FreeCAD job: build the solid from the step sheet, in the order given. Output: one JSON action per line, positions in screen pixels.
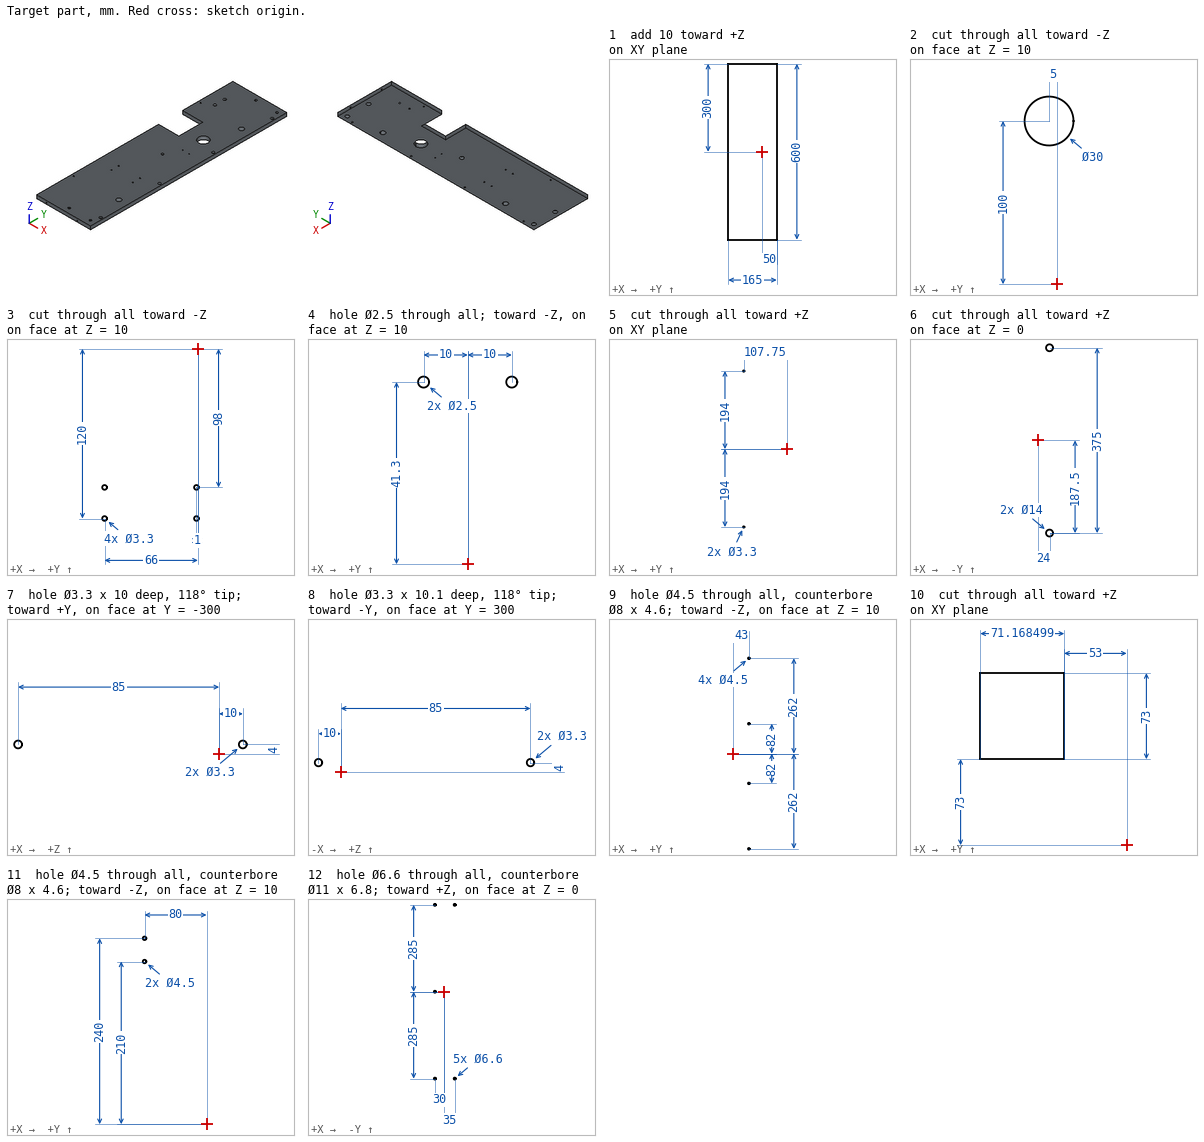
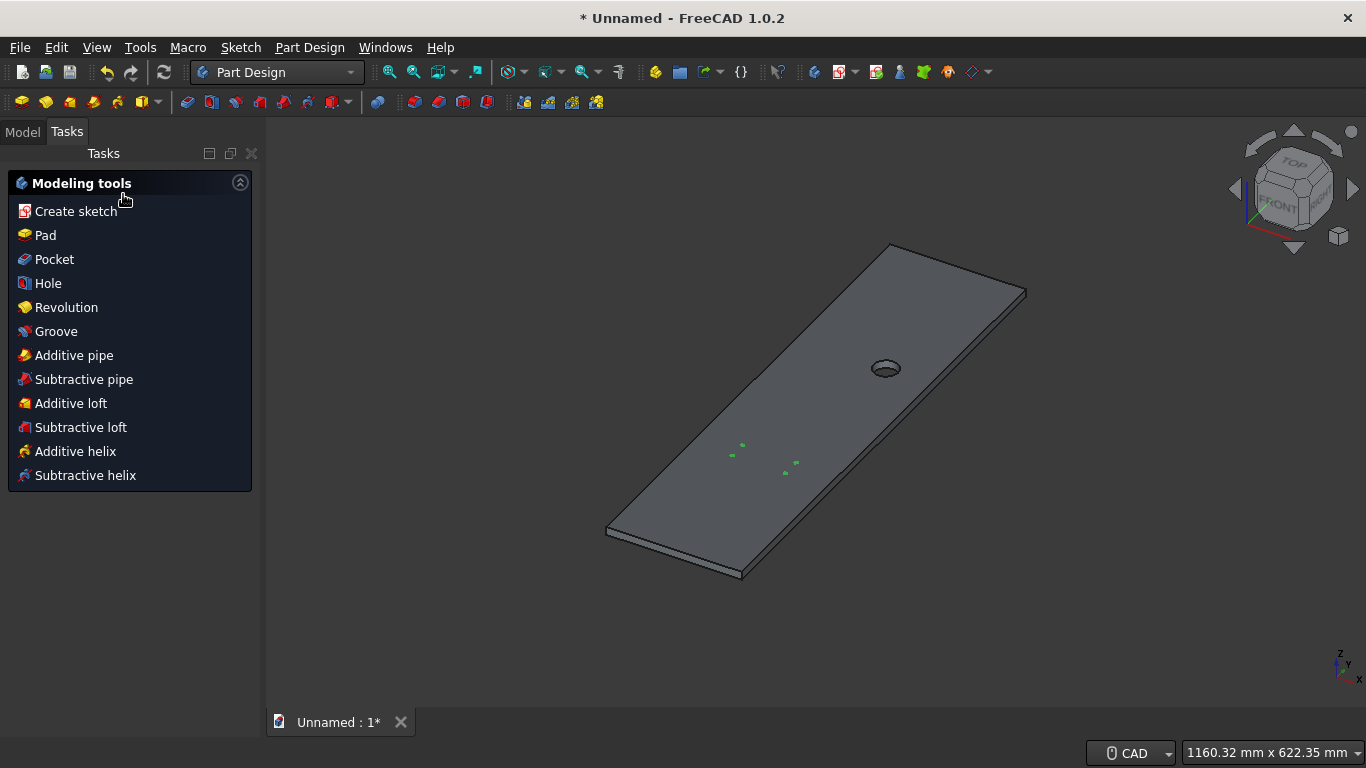
{"action": "left_click", "coordinate": [188, 102]}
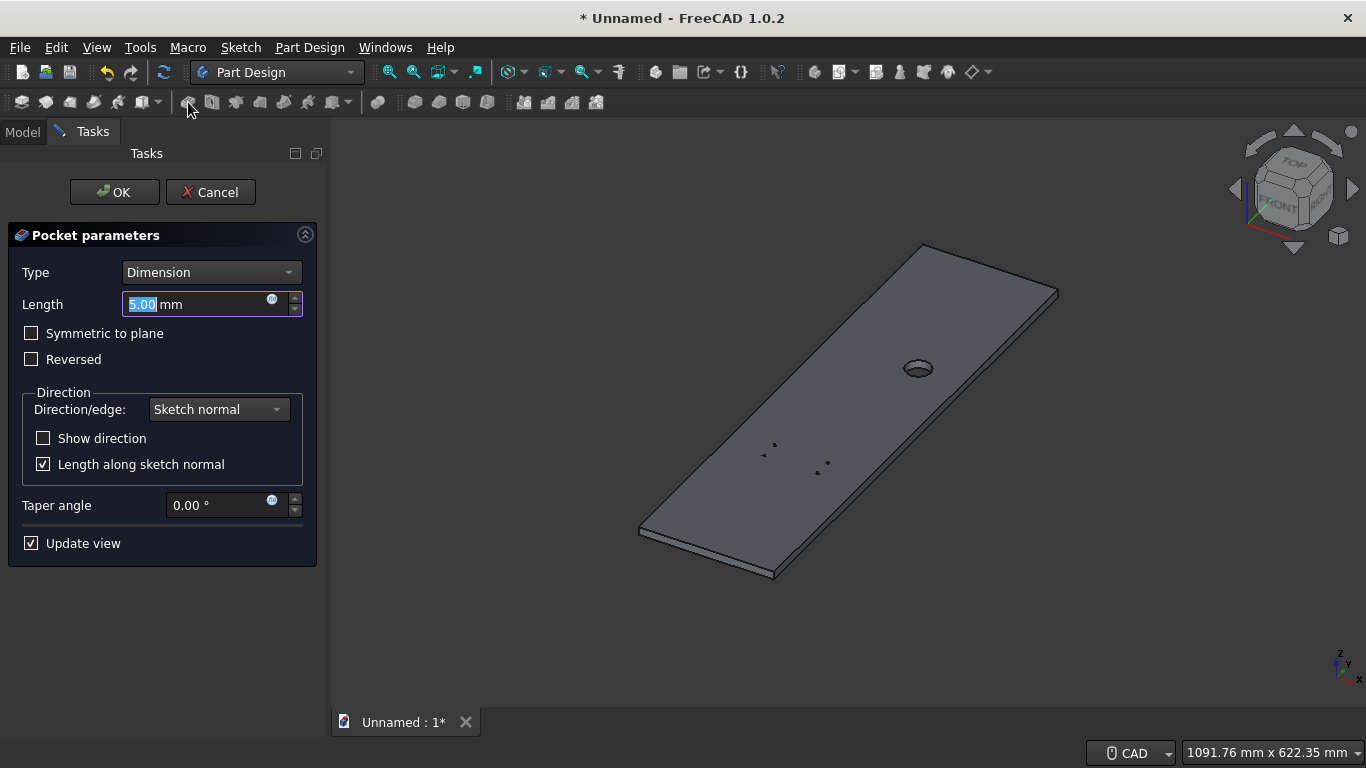
{"action": "left_click", "coordinate": [212, 272]}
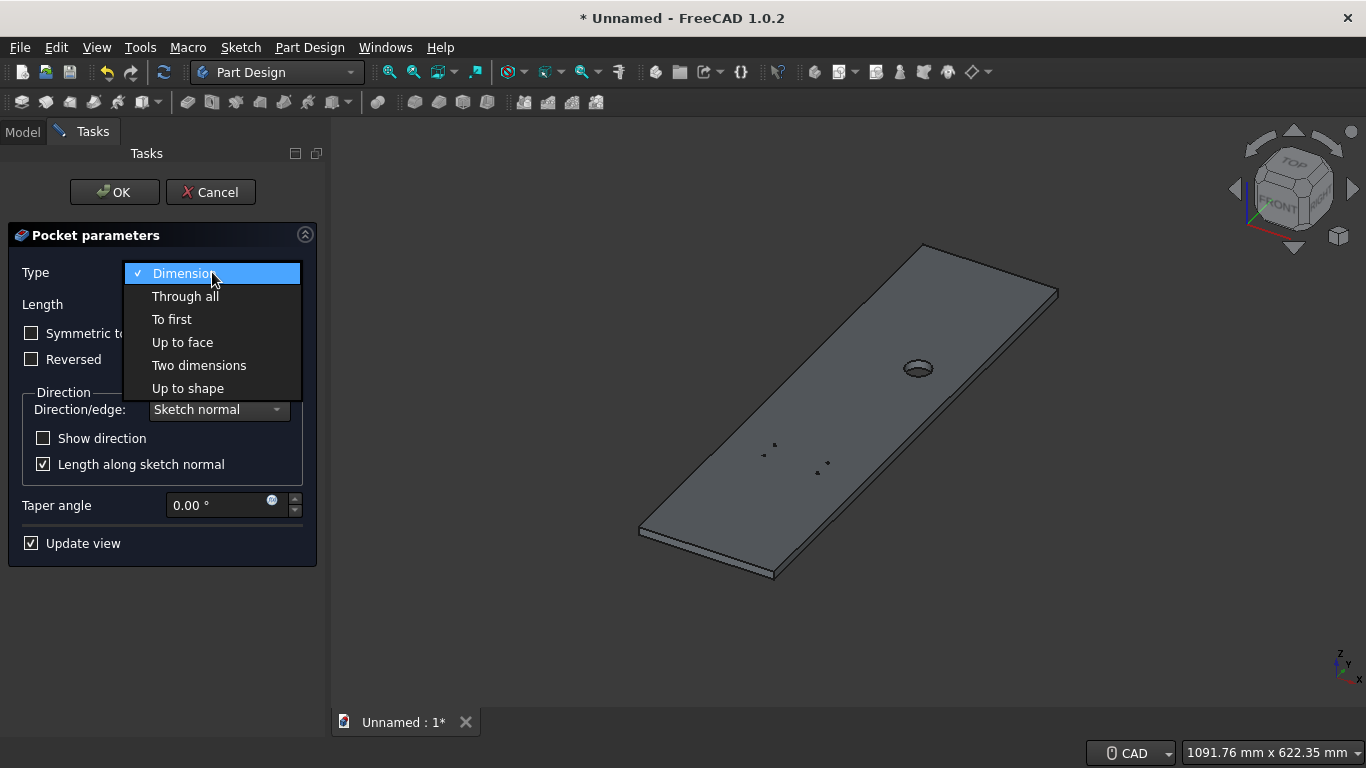
{"action": "left_click", "coordinate": [212, 296]}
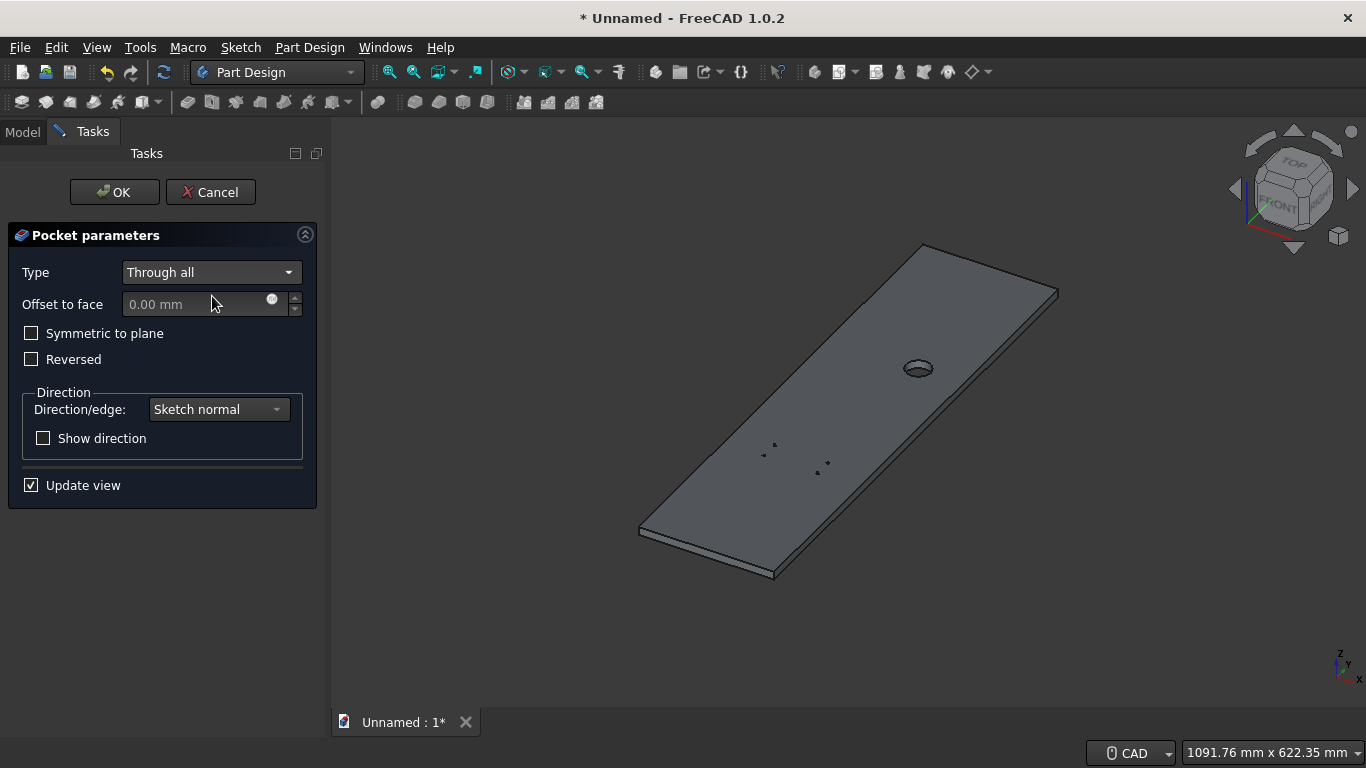
{"action": "left_click", "coordinate": [115, 192]}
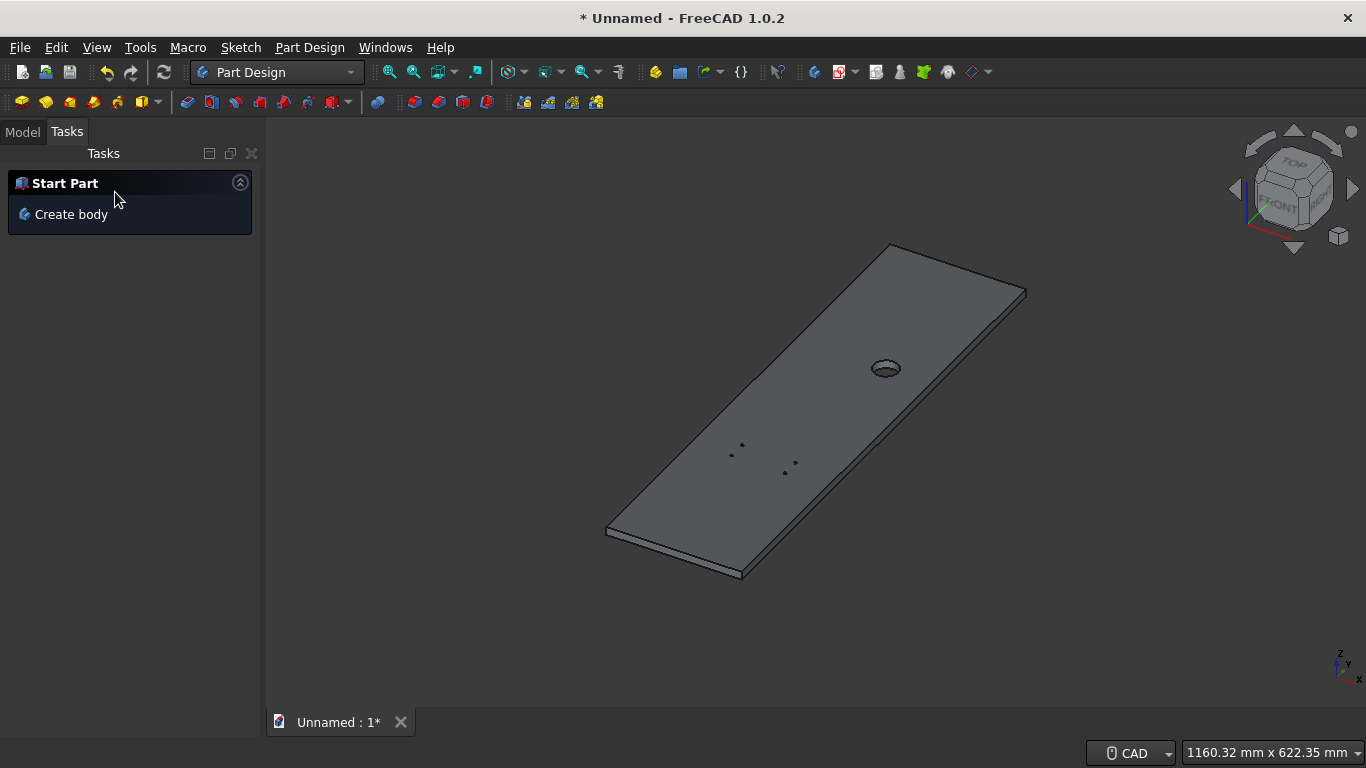
{"action": "left_click", "coordinate": [816, 407]}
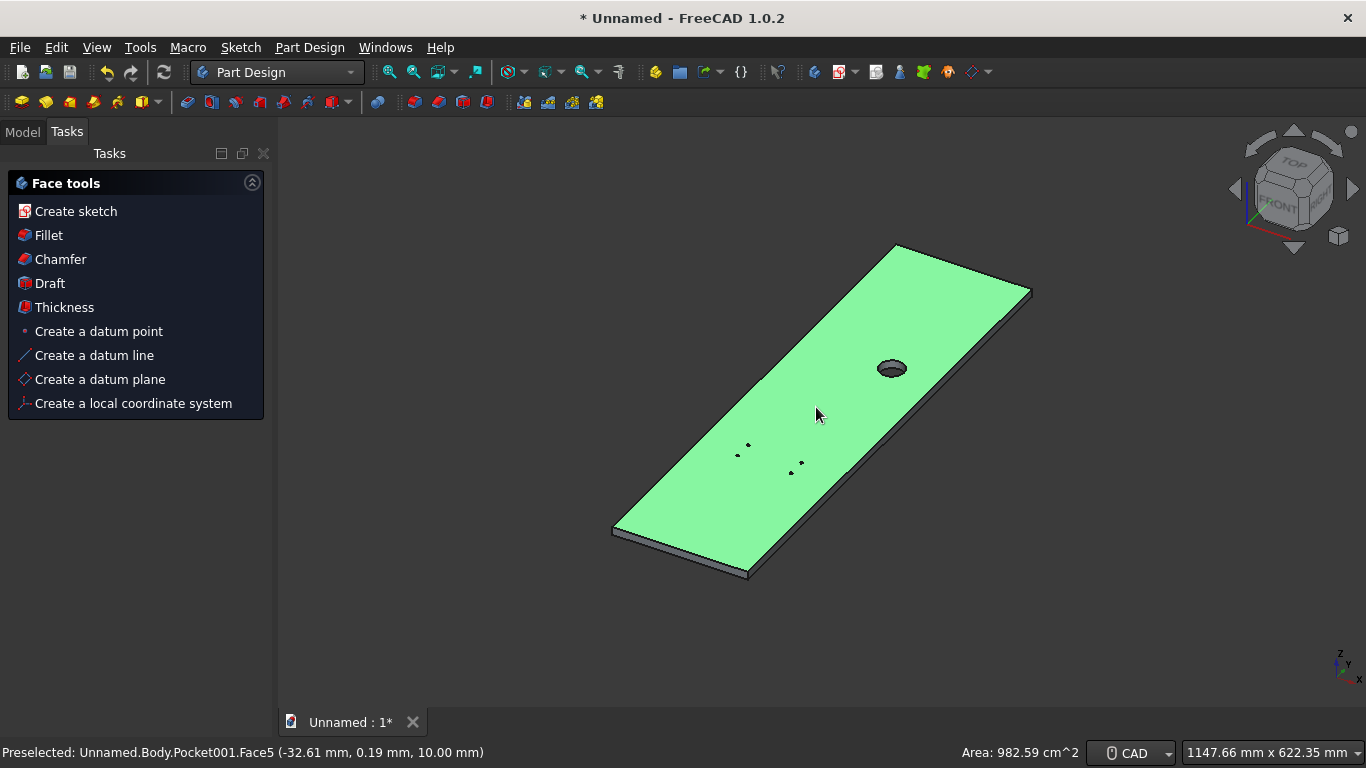
{"action": "left_click", "coordinate": [840, 72]}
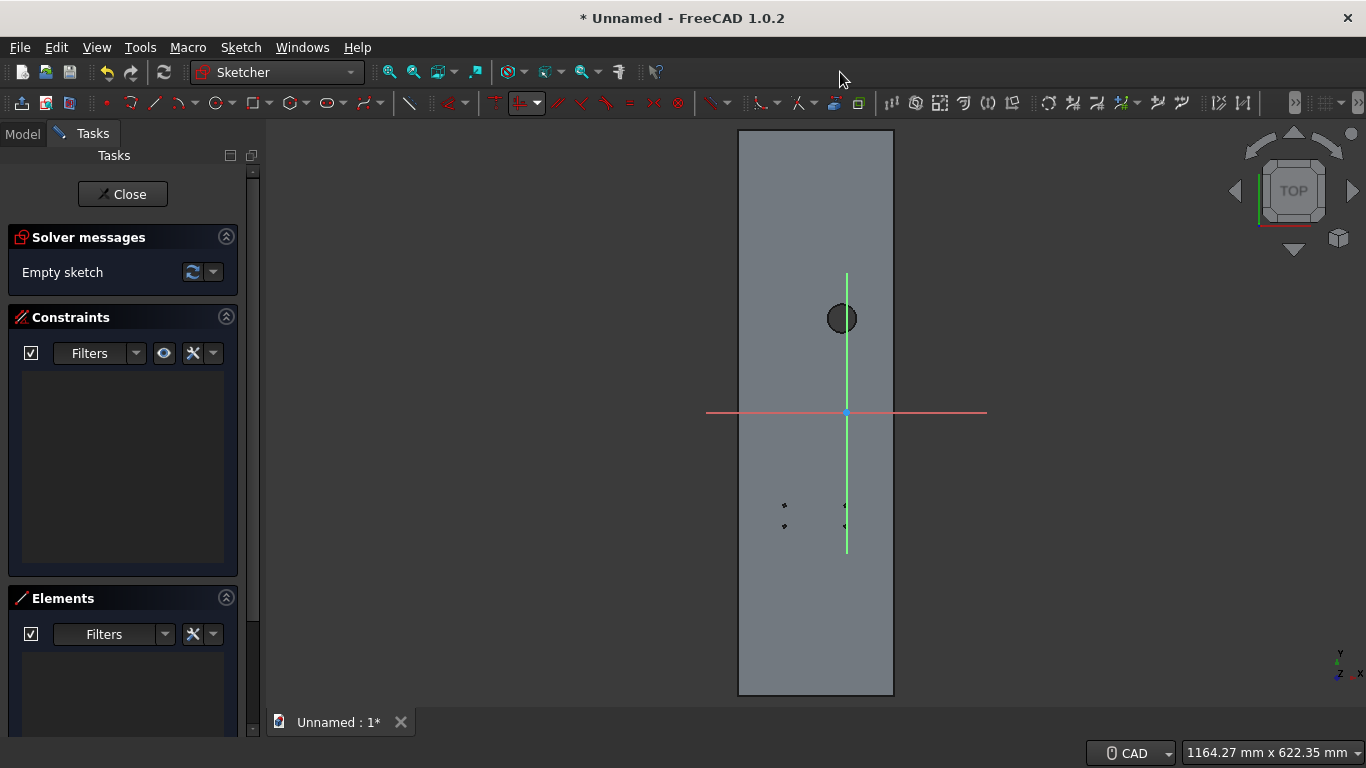
{"action": "scroll", "coordinate": [859, 390], "scroll_direction": "up", "scroll_amount": 11}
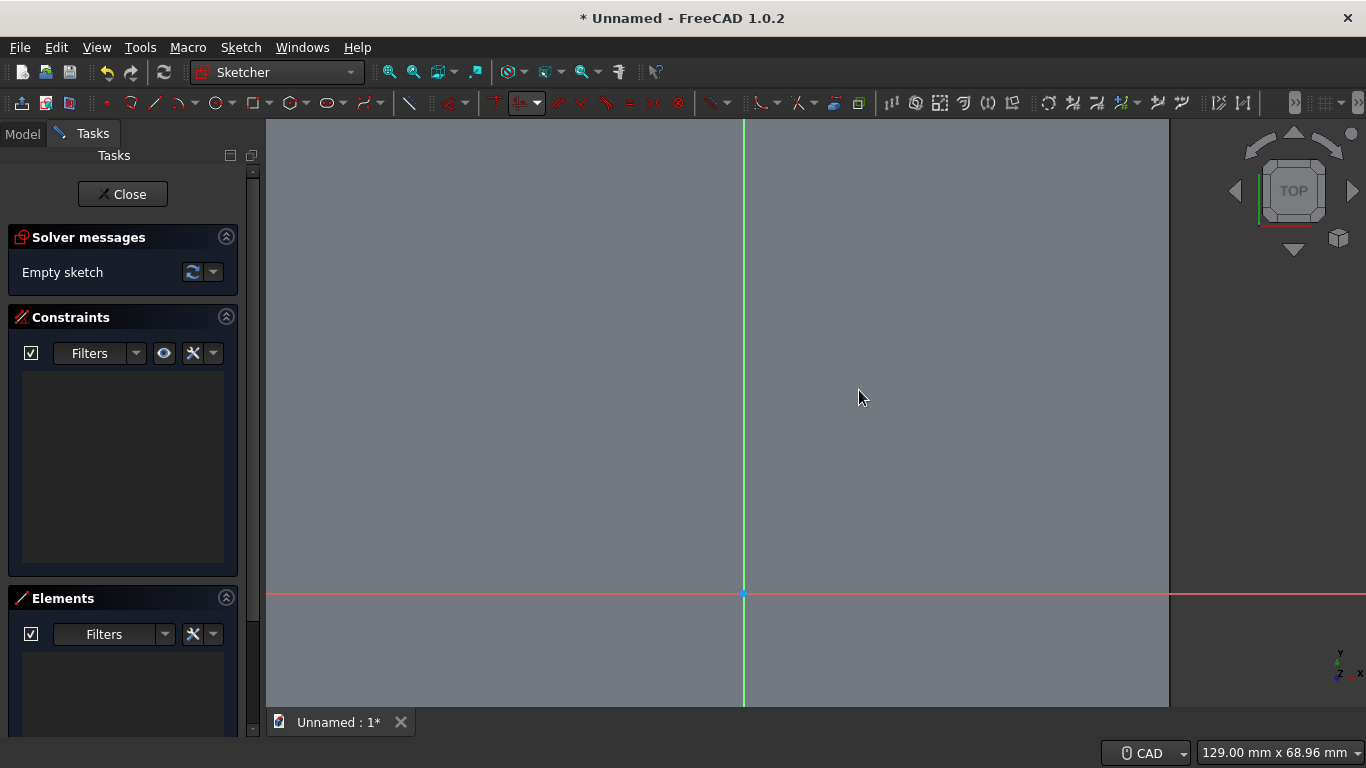
{"action": "left_click", "coordinate": [216, 104]}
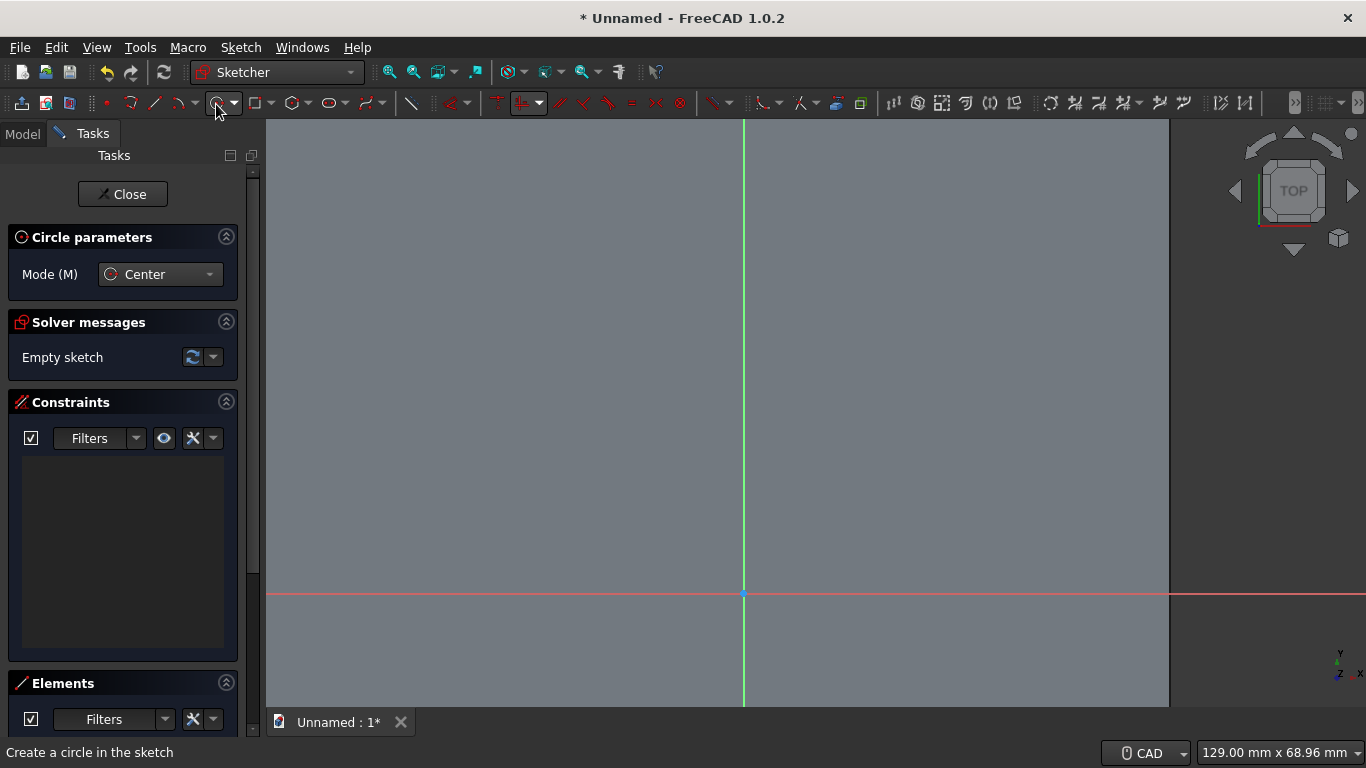
{"action": "scroll", "coordinate": [658, 242], "scroll_direction": "up", "scroll_amount": 4}